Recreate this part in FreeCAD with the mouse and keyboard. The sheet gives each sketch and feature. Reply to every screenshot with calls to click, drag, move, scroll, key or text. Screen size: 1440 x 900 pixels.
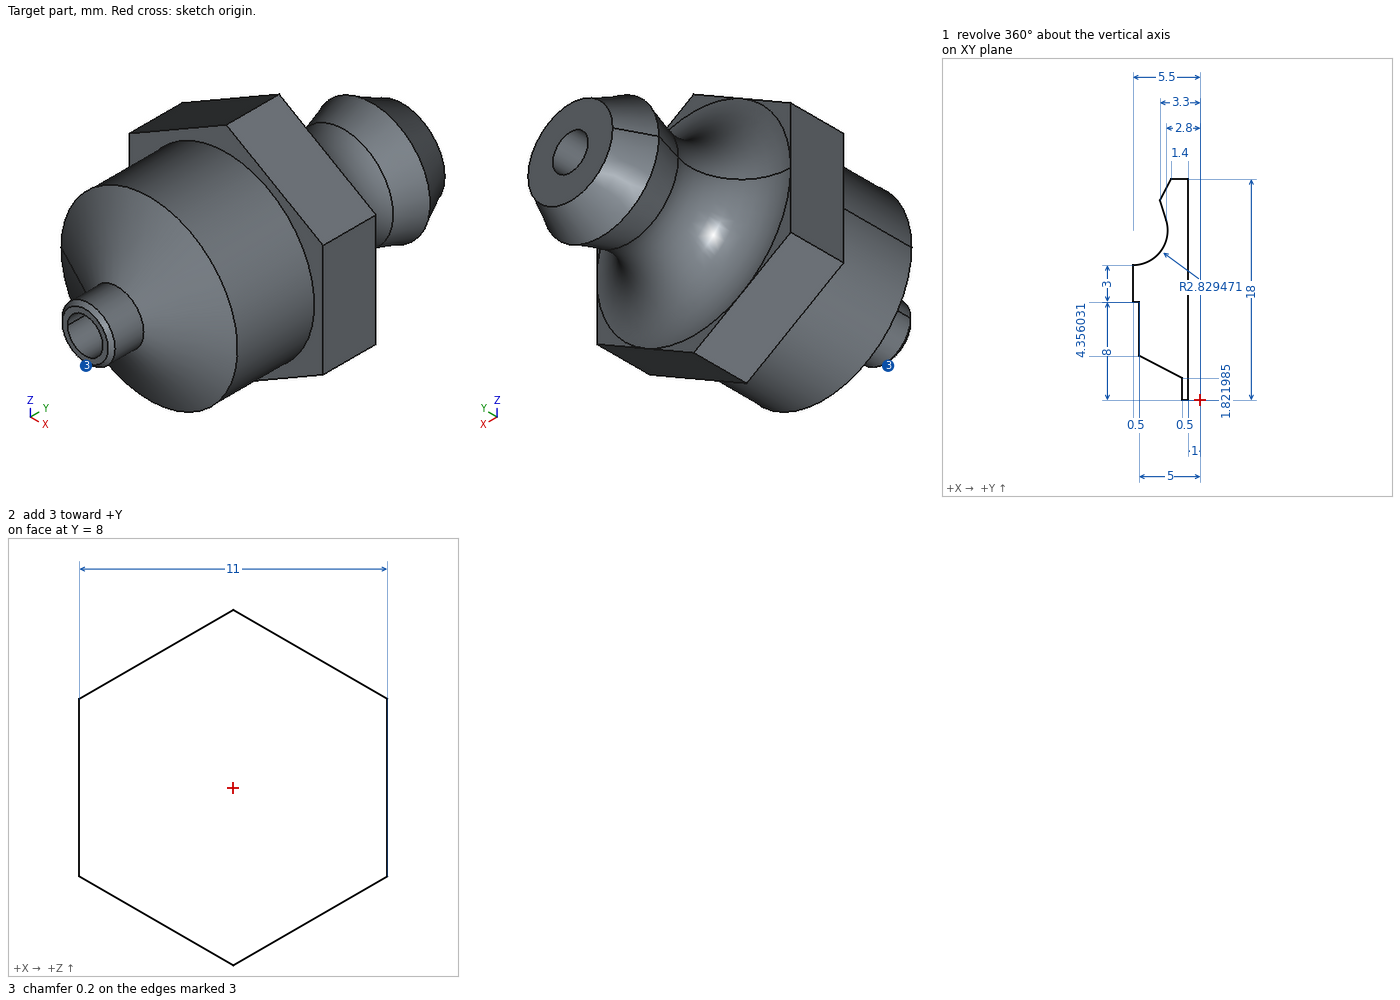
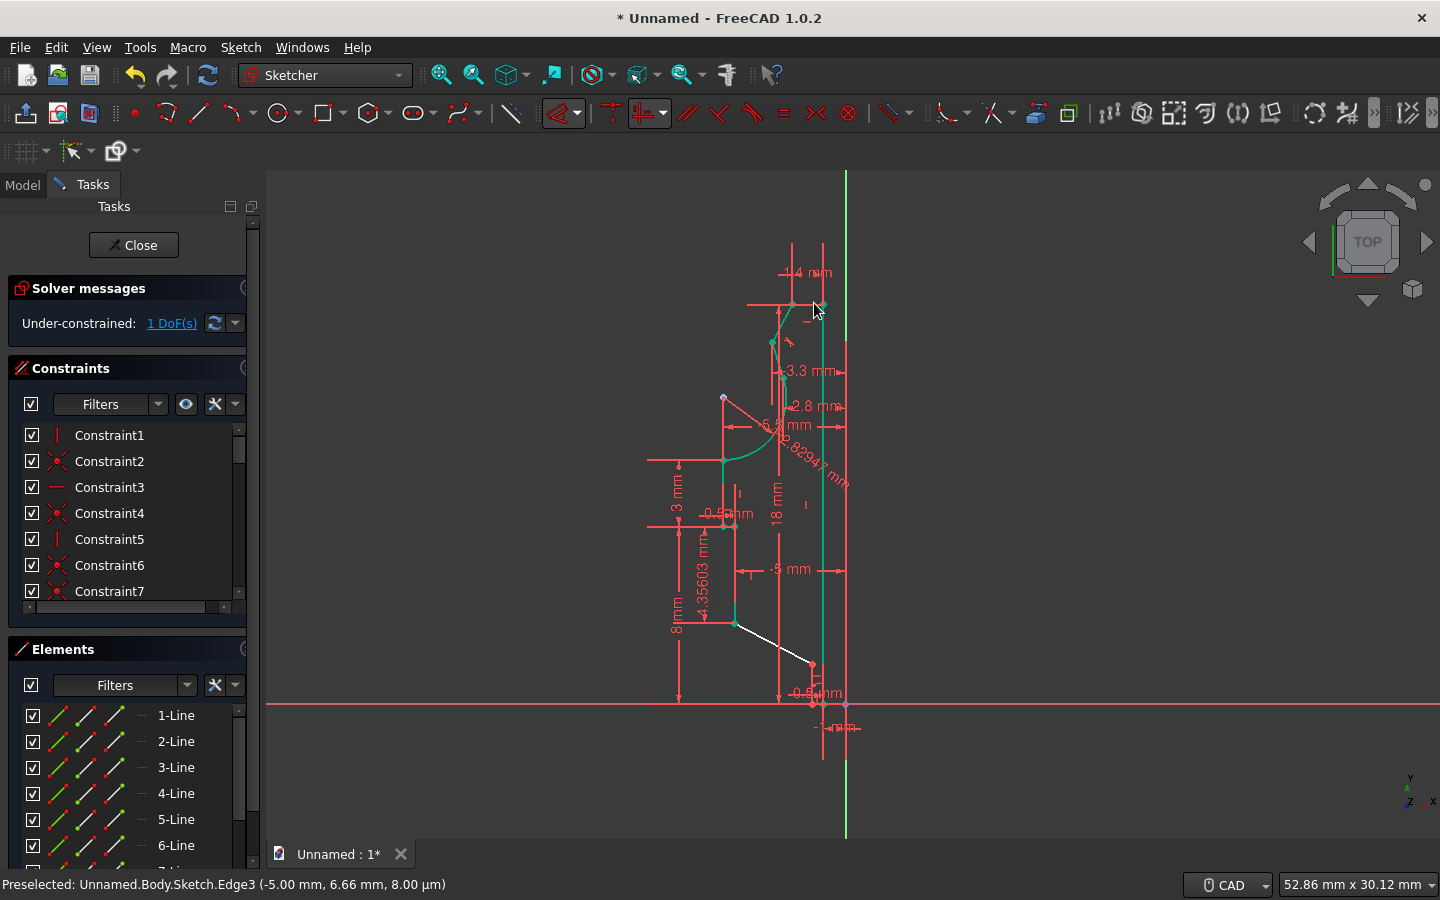
scroll(812, 676, up, 2)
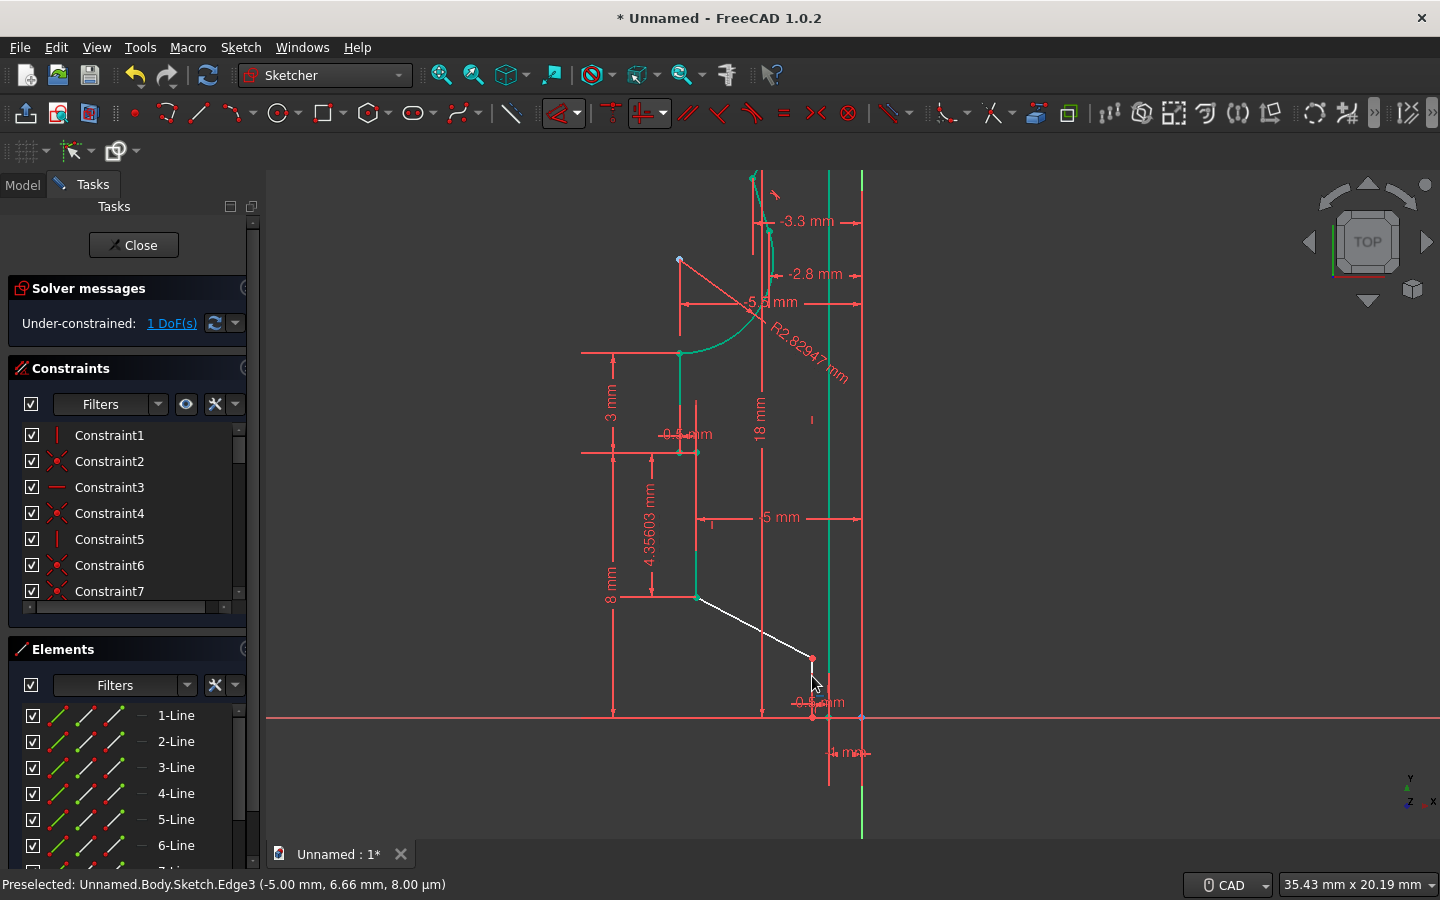
click(812, 676)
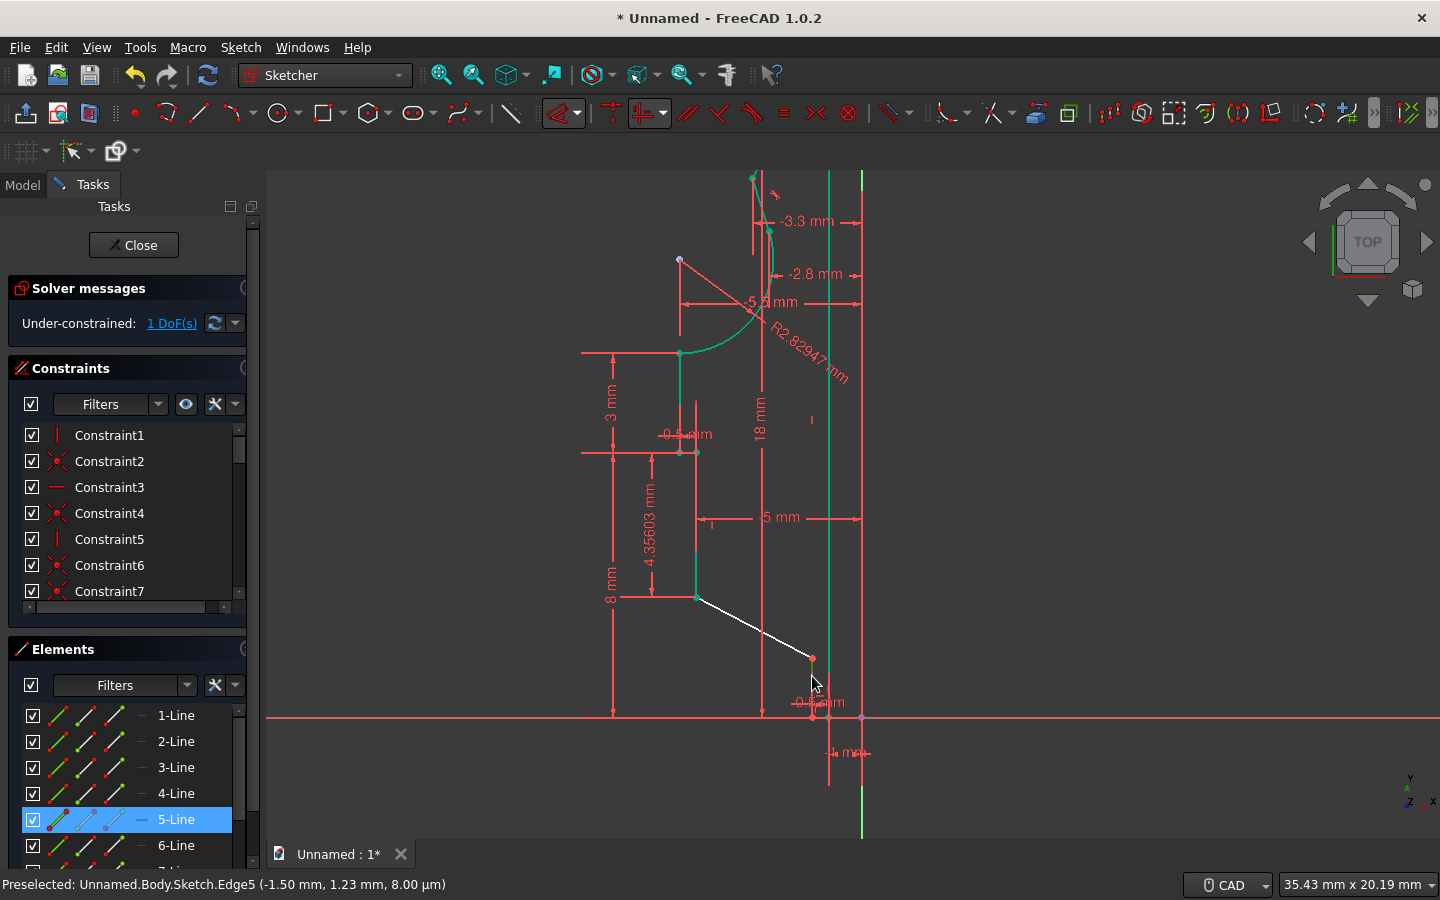
click(580, 114)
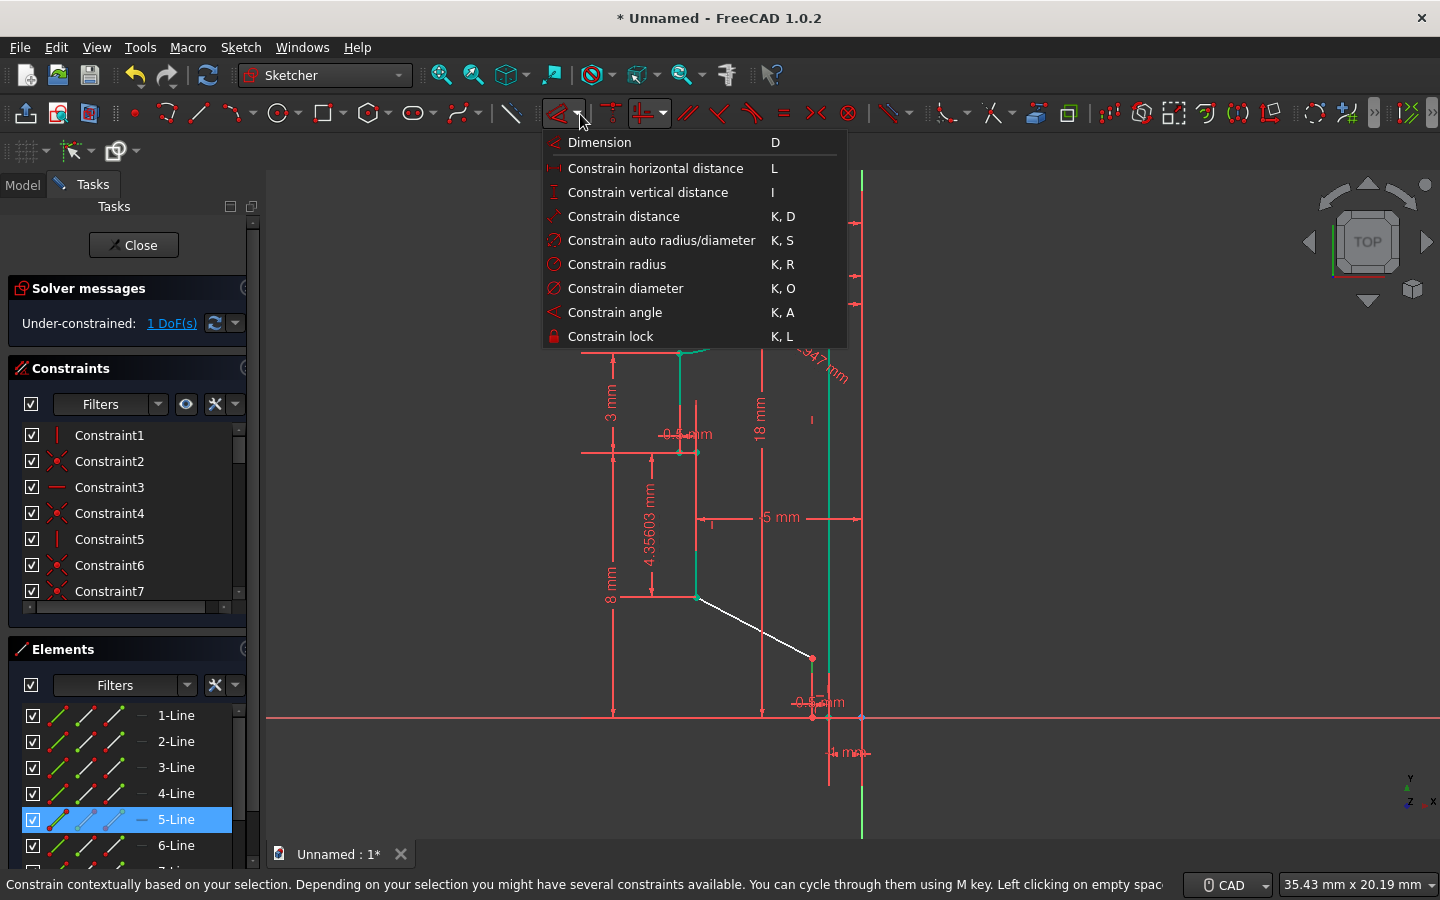
click(695, 192)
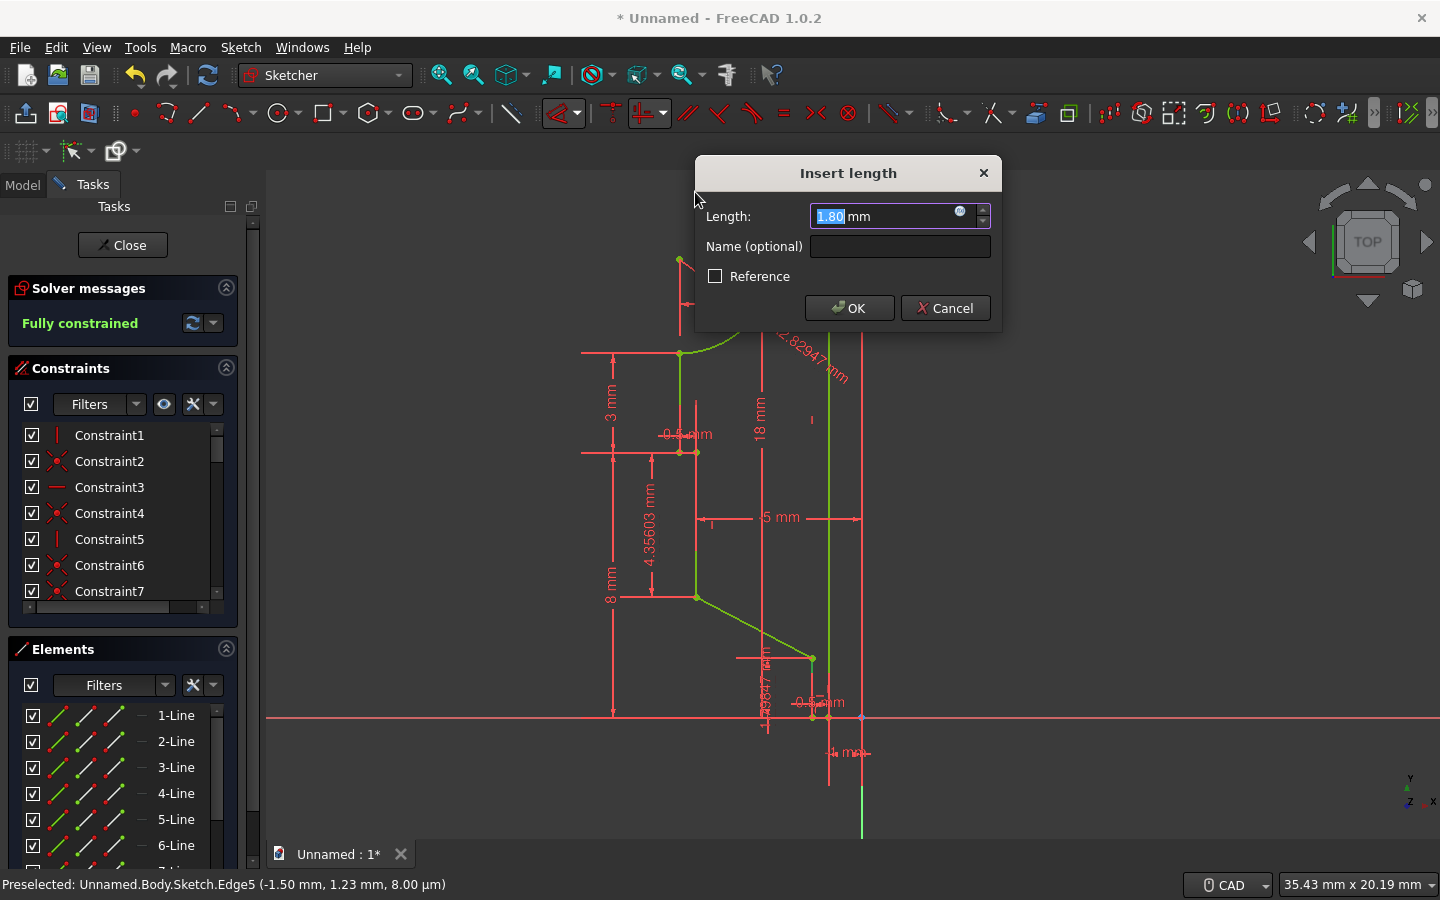
text(1.821985)
key(Return)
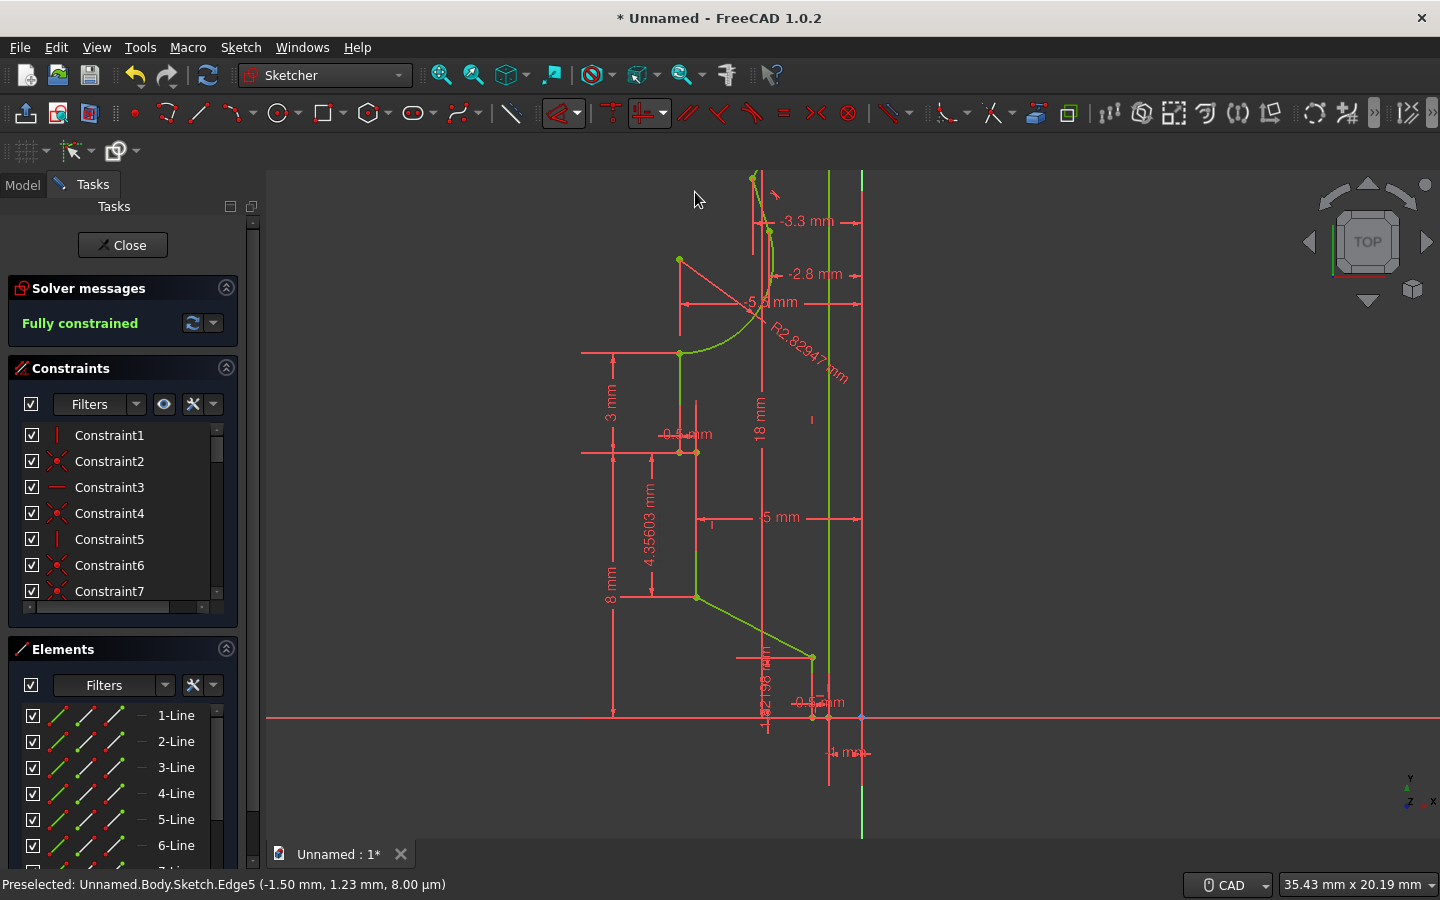
click(123, 245)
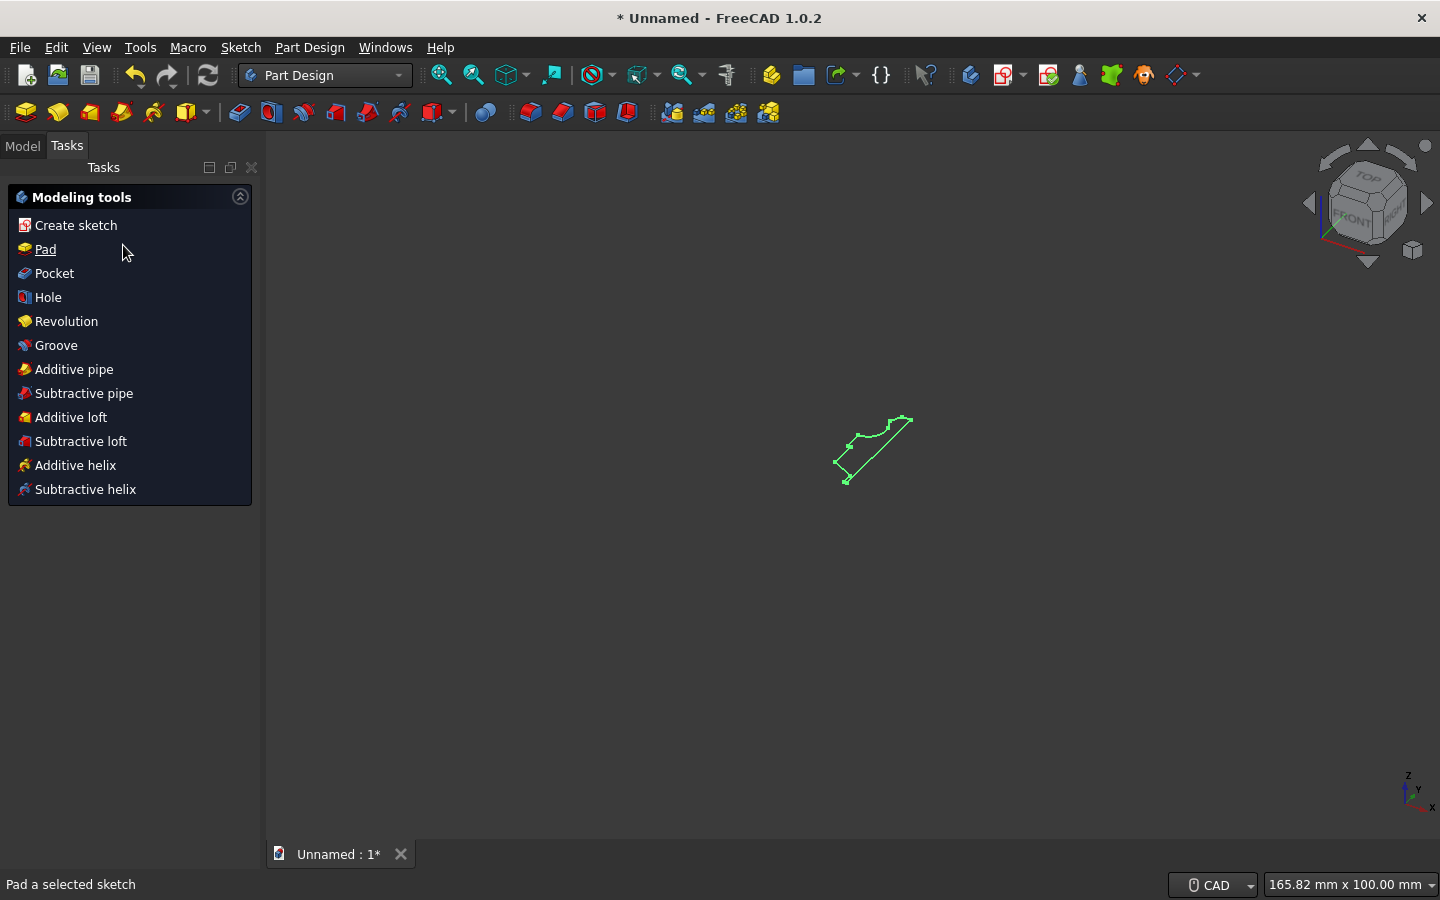
click(58, 112)